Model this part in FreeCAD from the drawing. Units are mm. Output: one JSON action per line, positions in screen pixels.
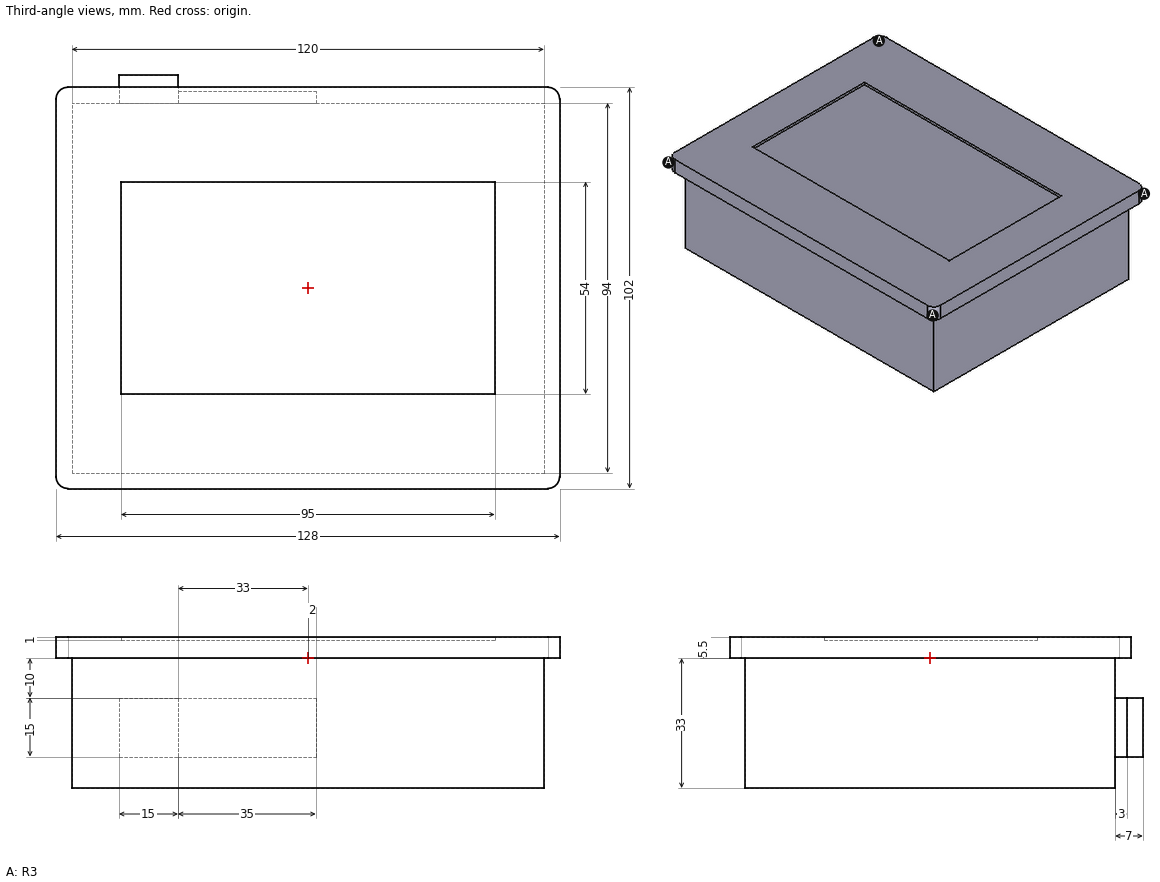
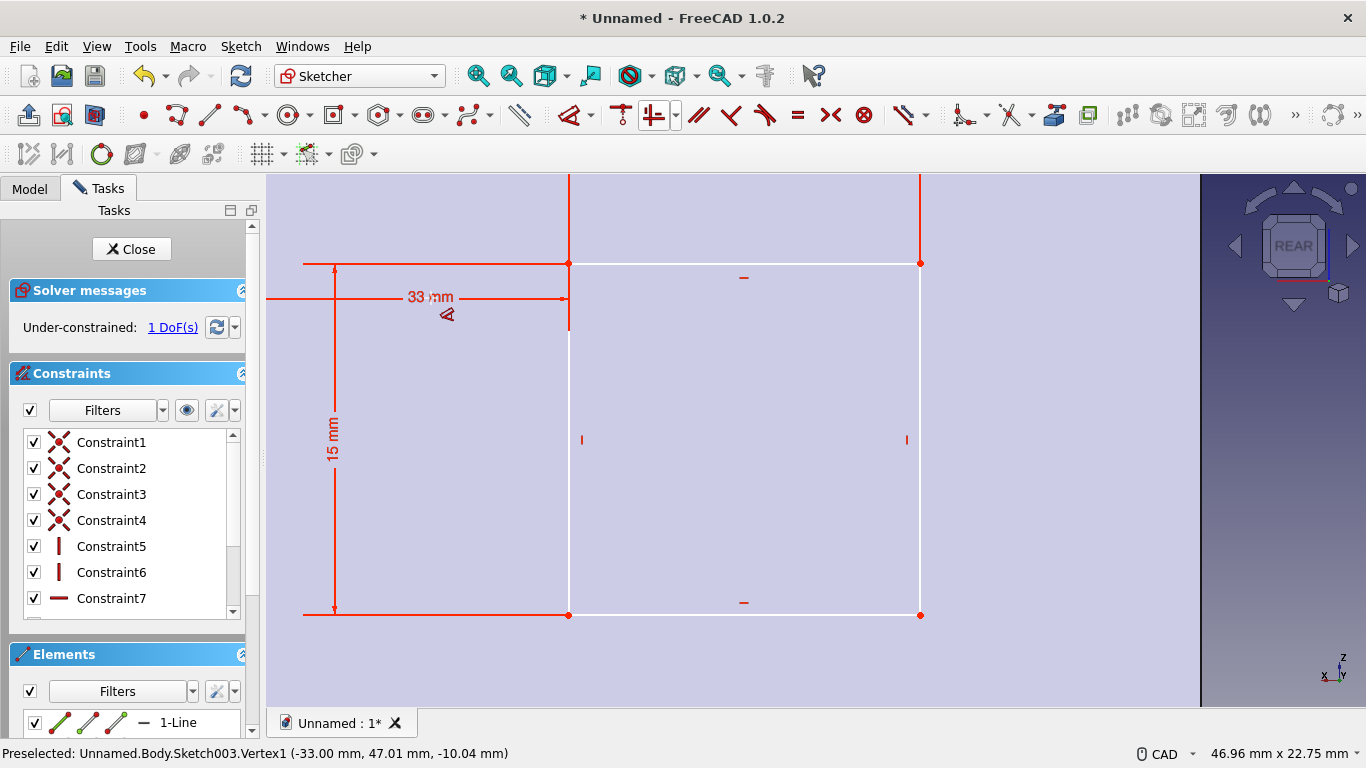
{"action": "left_click", "coordinate": [569, 264]}
{"action": "left_click", "coordinate": [603, 233]}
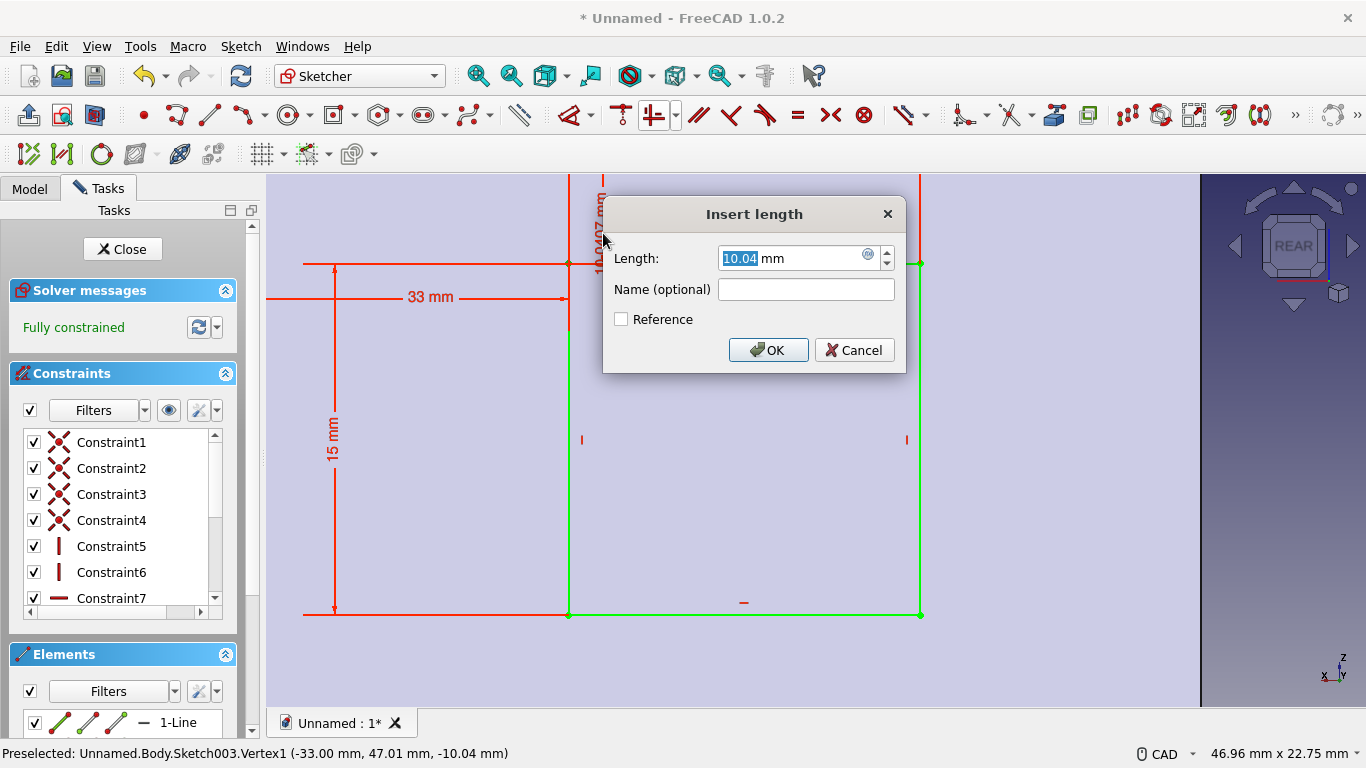
{"action": "type", "text": "10"}
{"action": "key", "text": "Return"}
{"action": "key", "text": "Escape"}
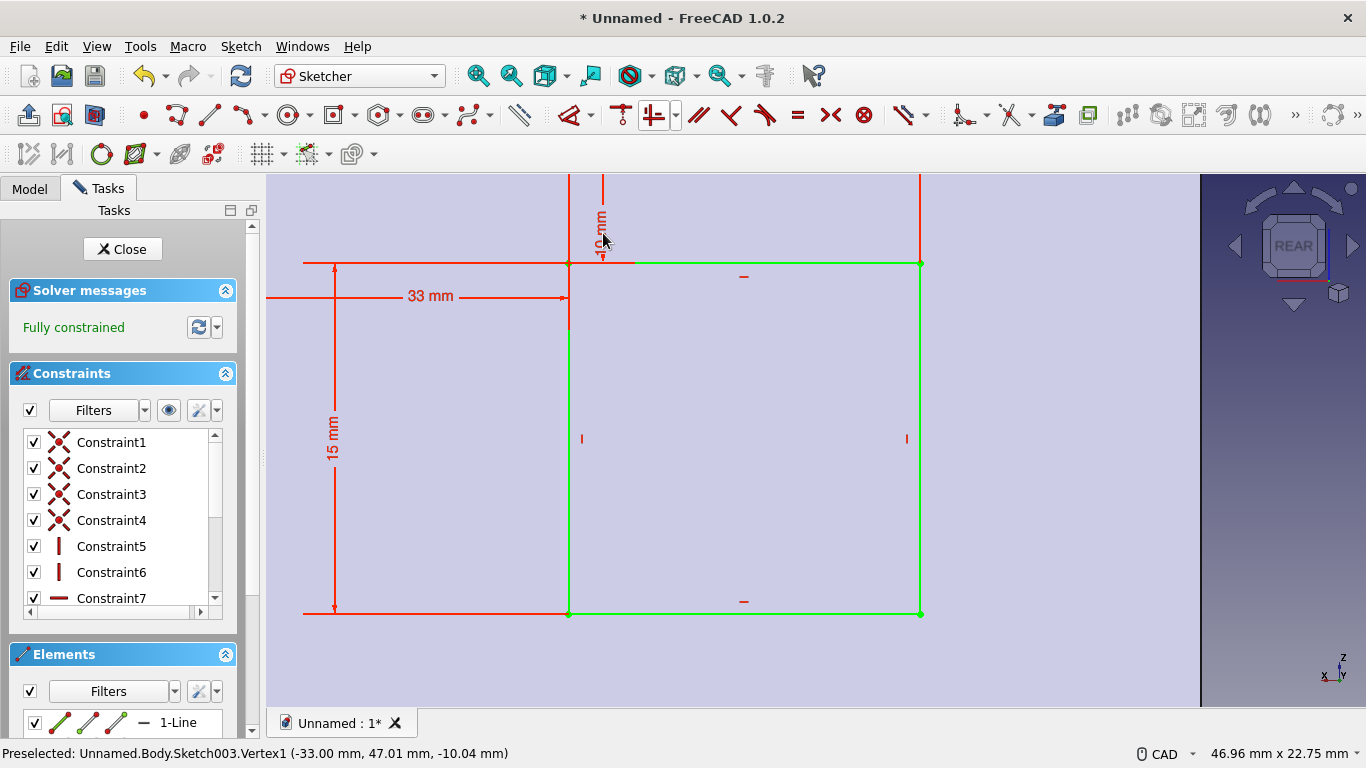
{"action": "left_click", "coordinate": [123, 249]}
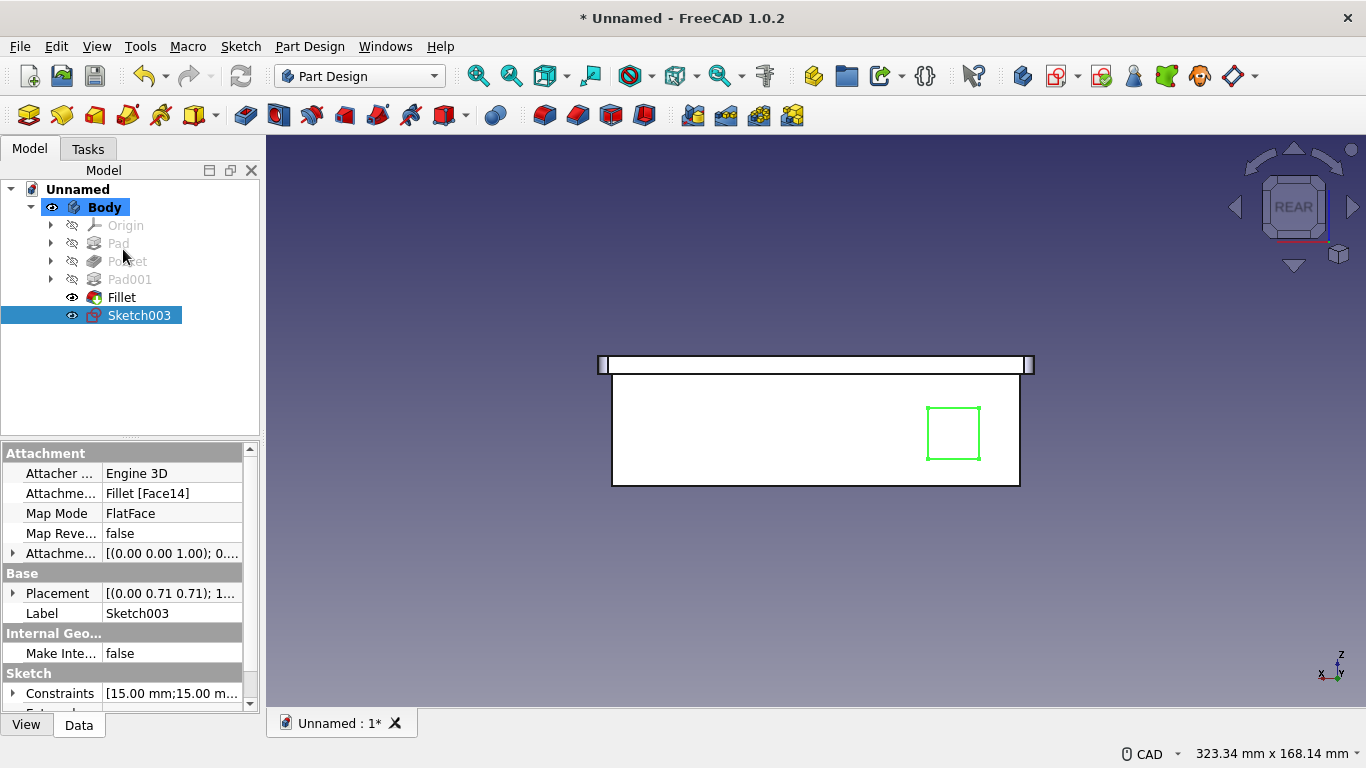
{"action": "left_click", "coordinate": [29, 116]}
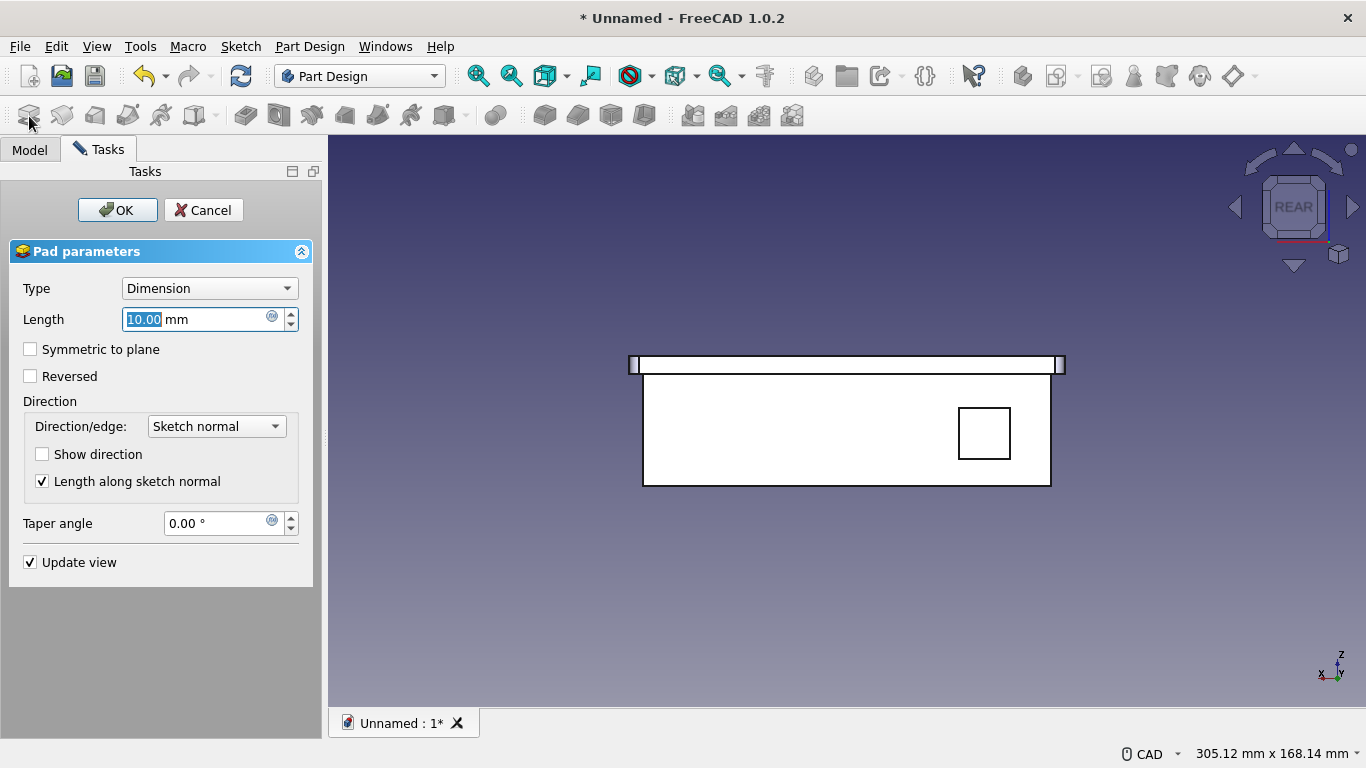
{"action": "type", "text": "7"}
{"action": "key", "text": "Tab"}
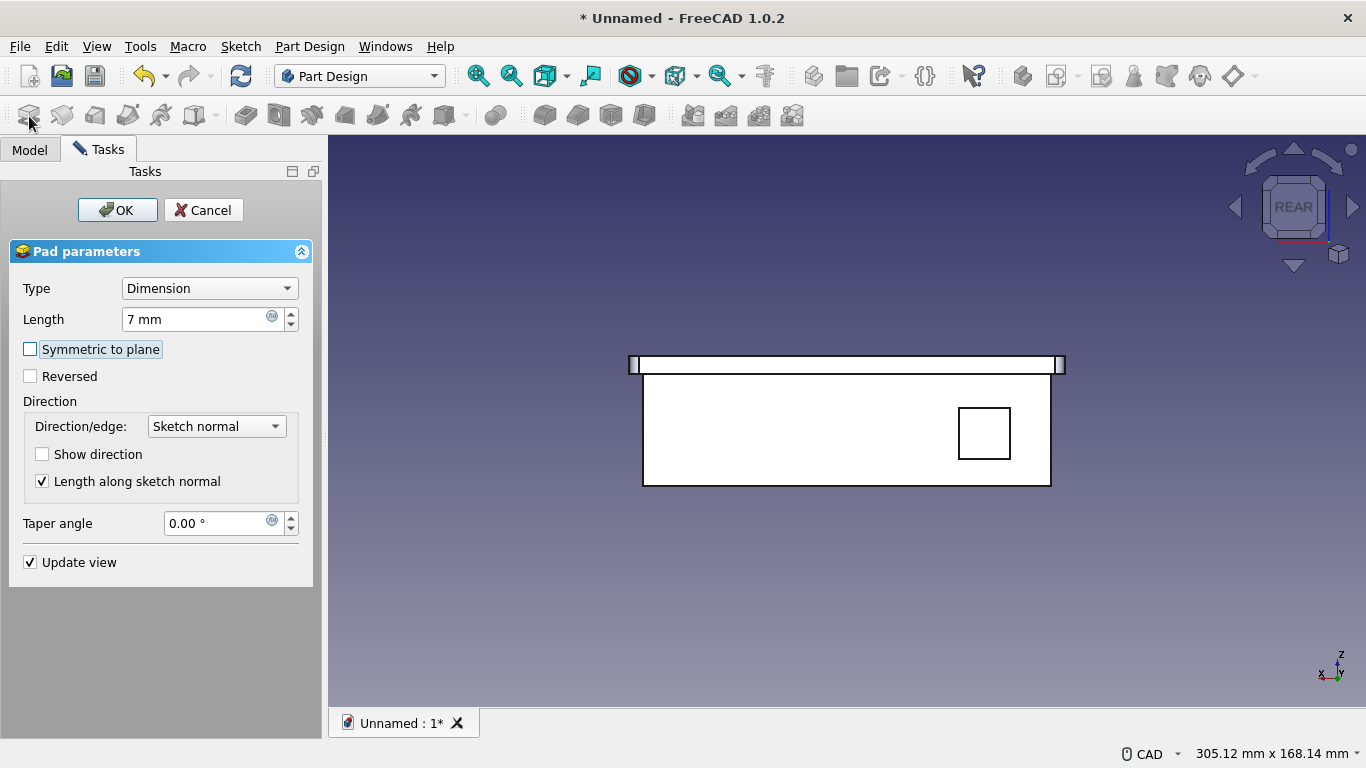
{"action": "left_click", "coordinate": [118, 210]}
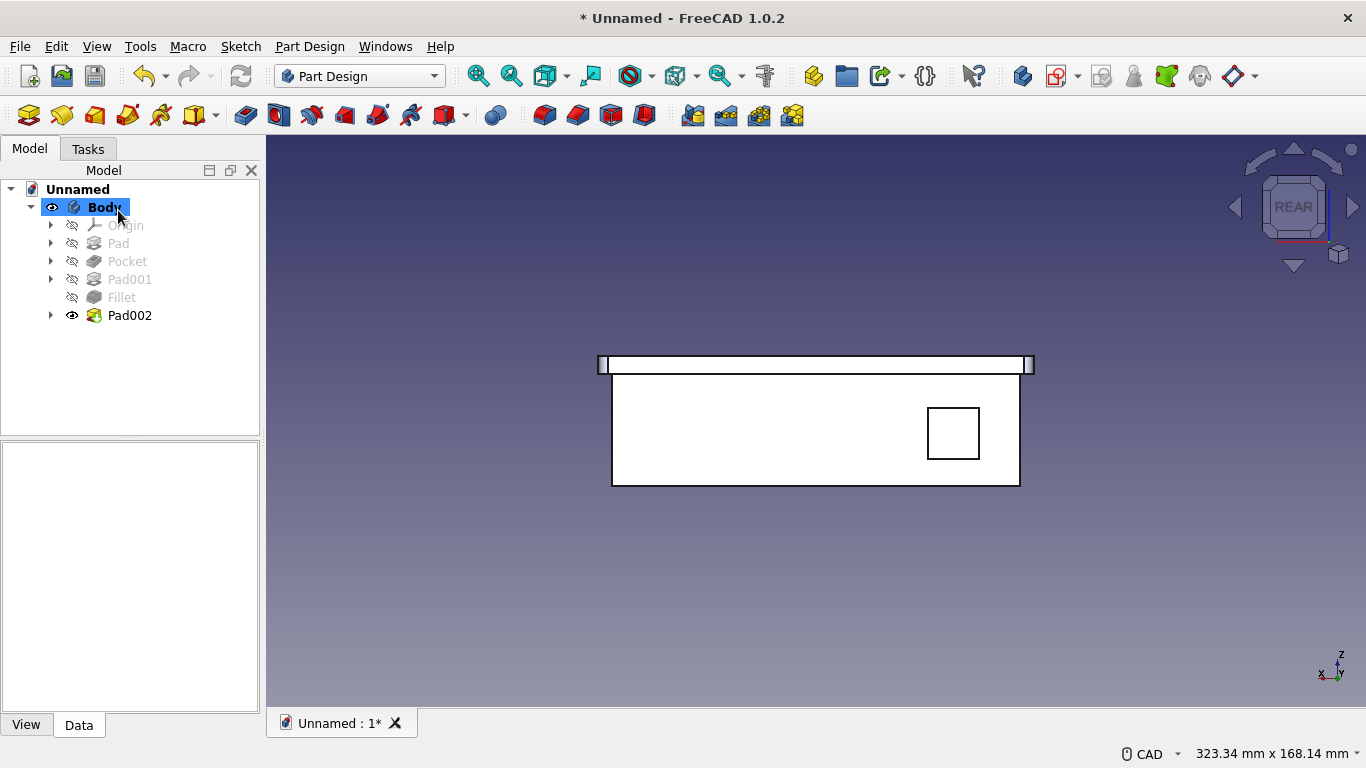
{"action": "key", "text": "v f"}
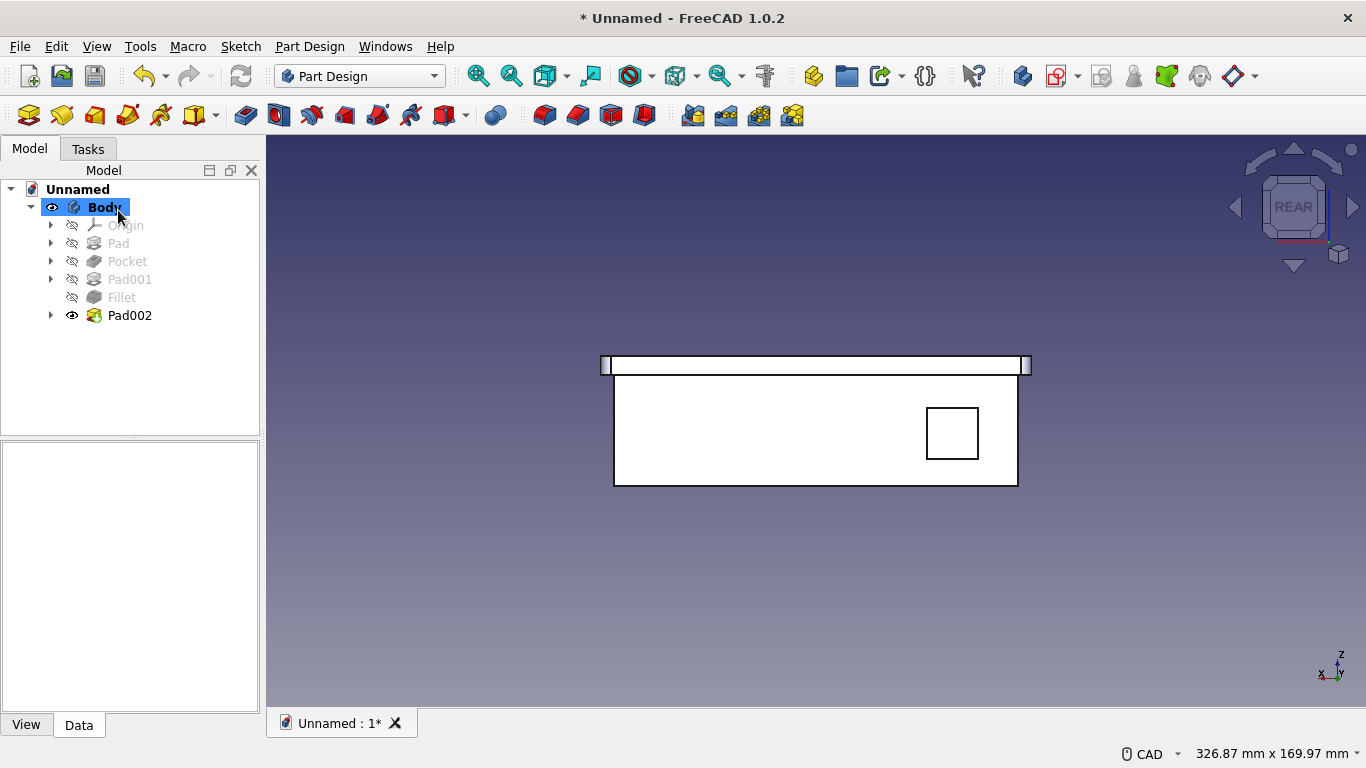
{"action": "left_click", "coordinate": [1023, 76]}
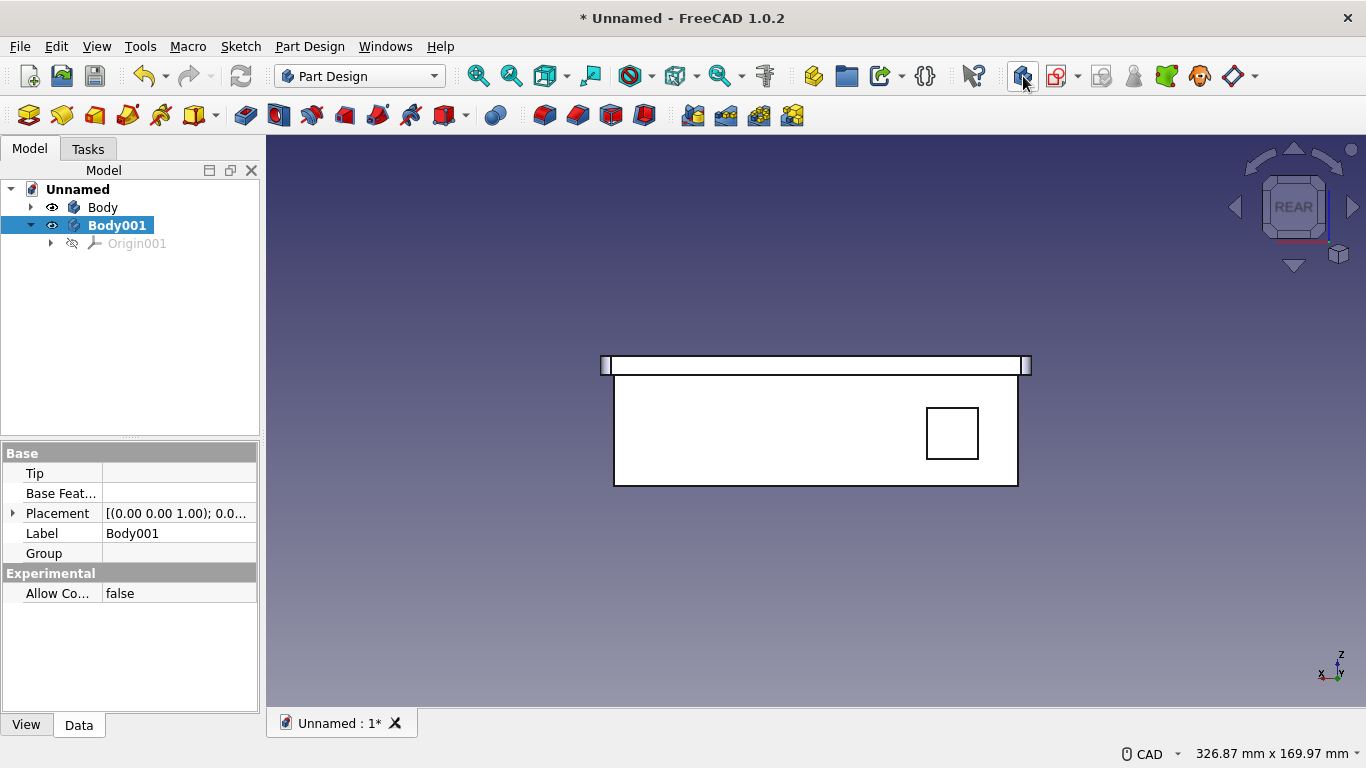
{"action": "left_click", "coordinate": [51, 243]}